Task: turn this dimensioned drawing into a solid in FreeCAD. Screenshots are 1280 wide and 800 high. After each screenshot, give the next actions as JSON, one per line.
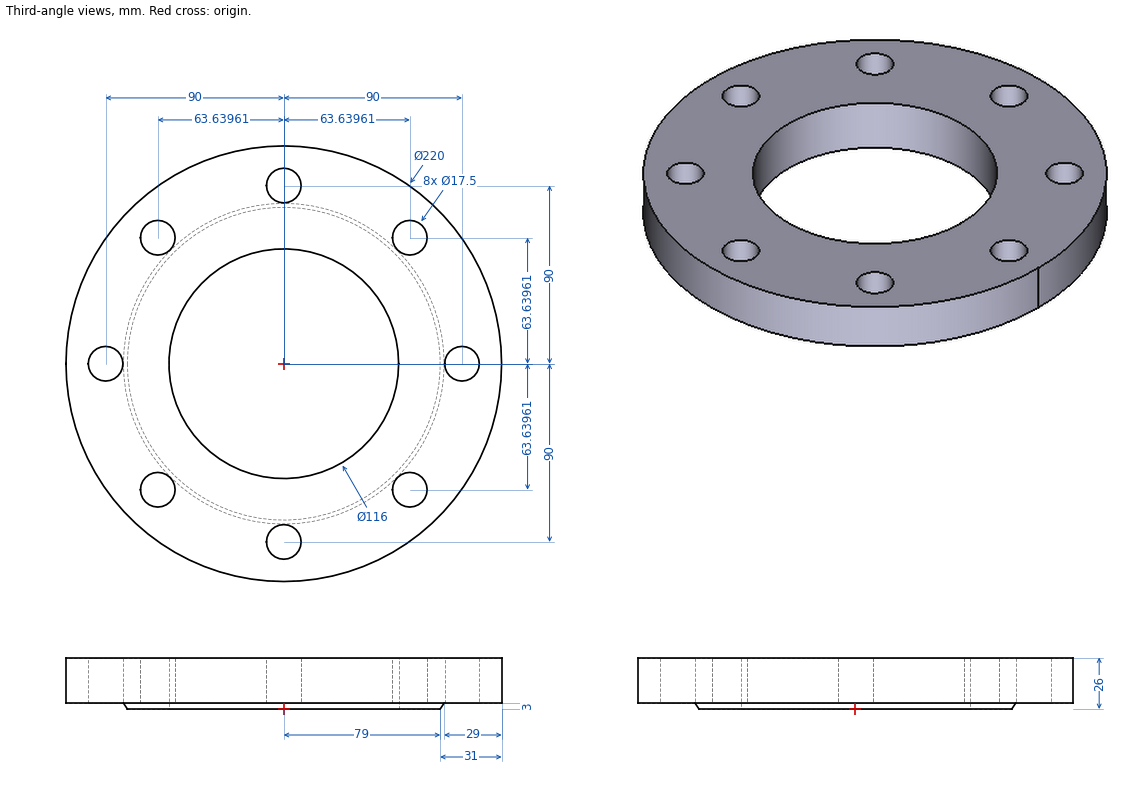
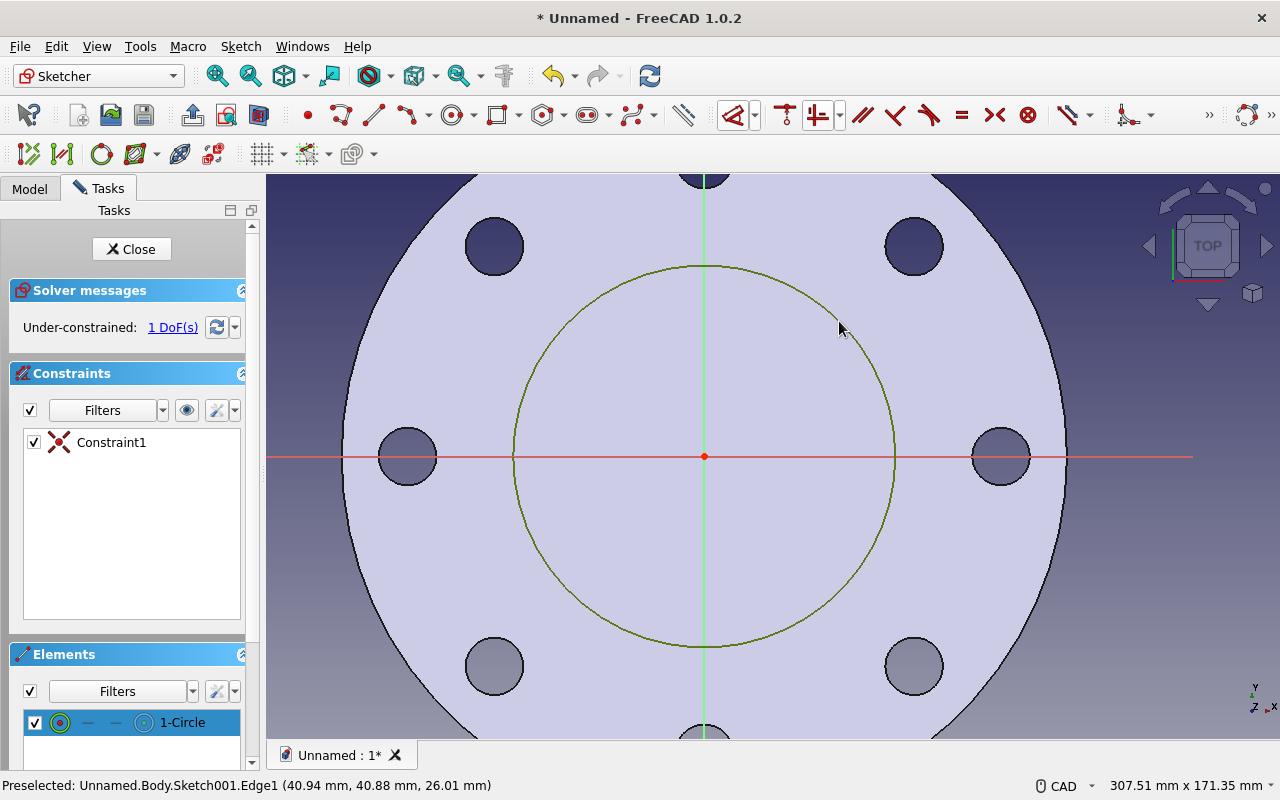
{"action": "left_click", "coordinate": [754, 116]}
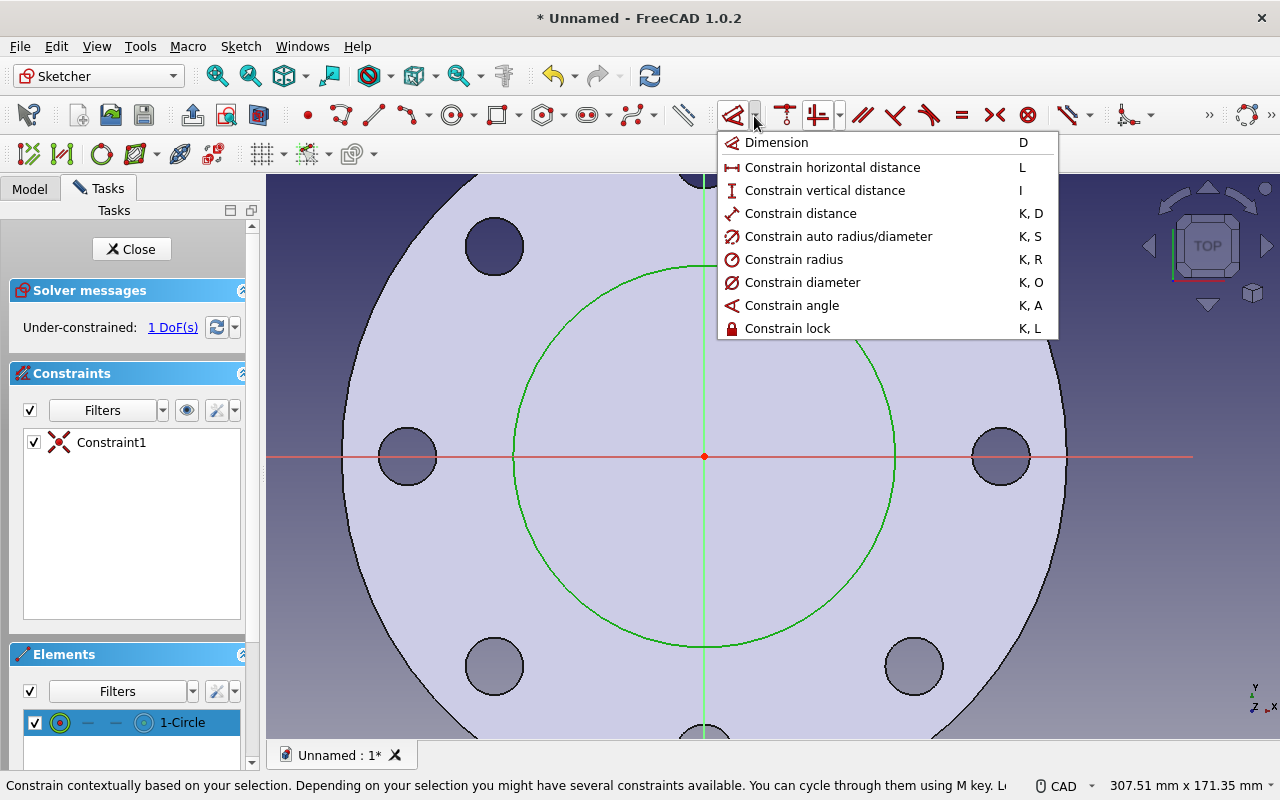
{"action": "left_click", "coordinate": [888, 282]}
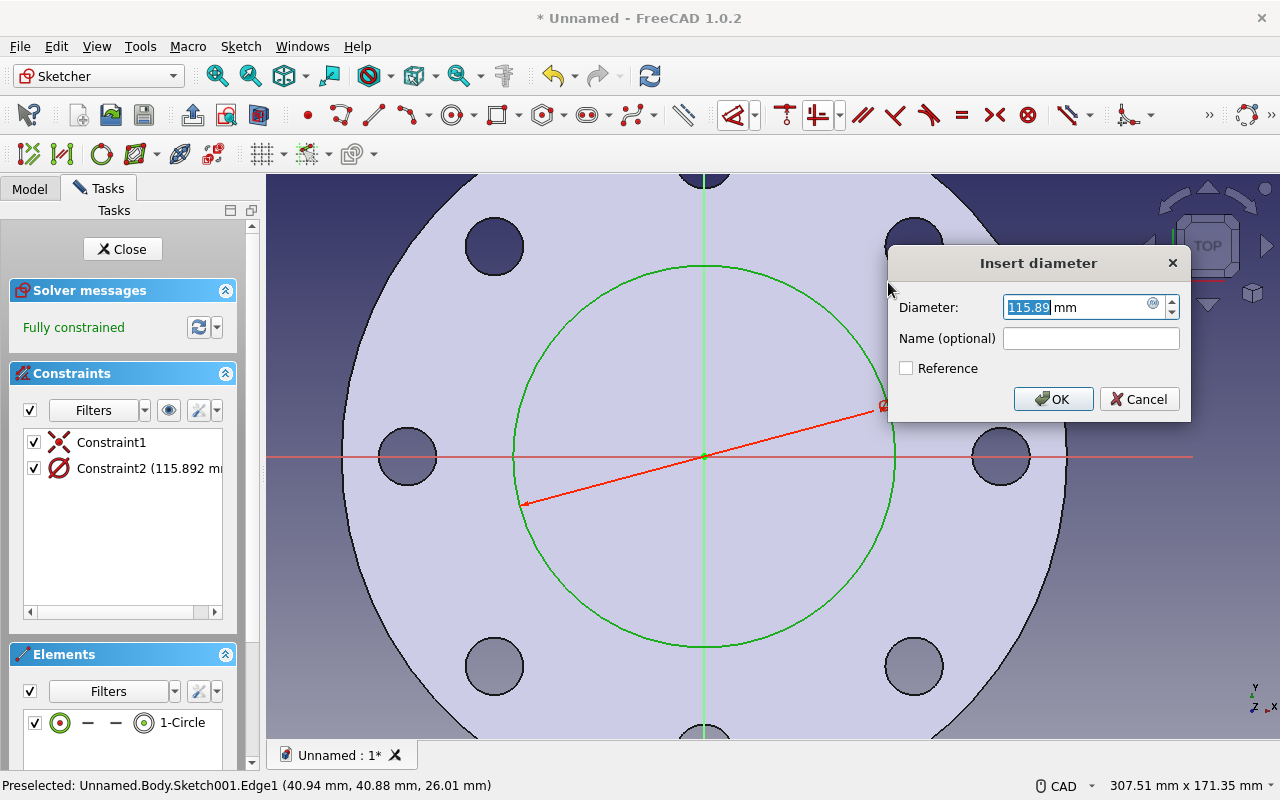
{"action": "type", "text": "116"}
{"action": "key", "text": "Return"}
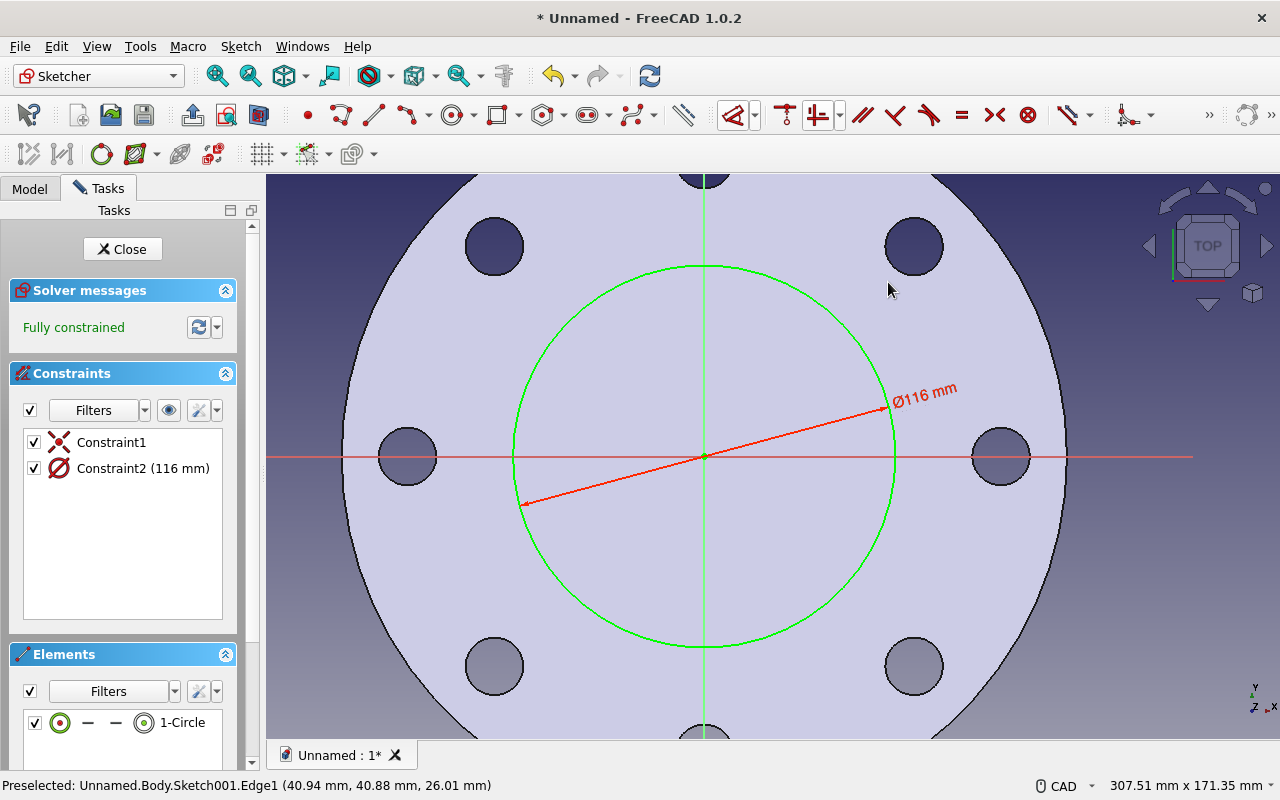
{"action": "left_click", "coordinate": [123, 249]}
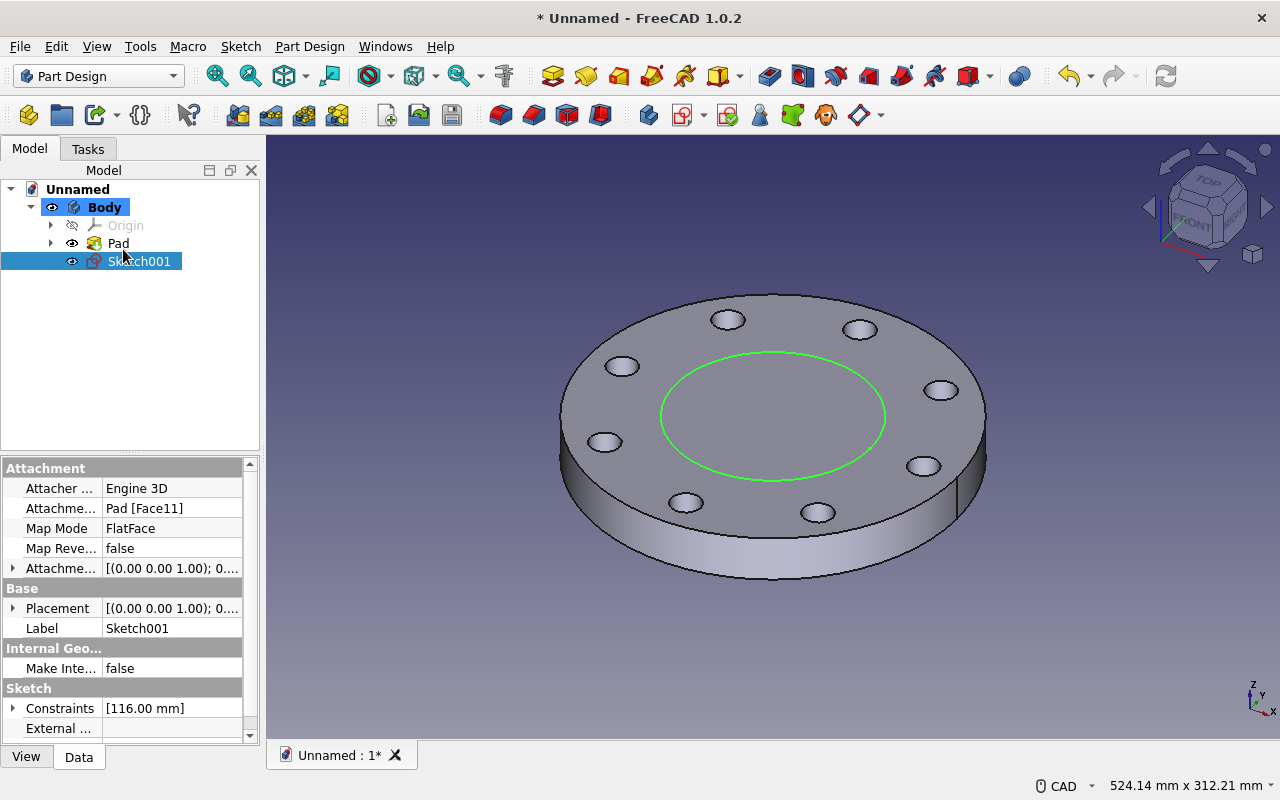
{"action": "left_click", "coordinate": [770, 76]}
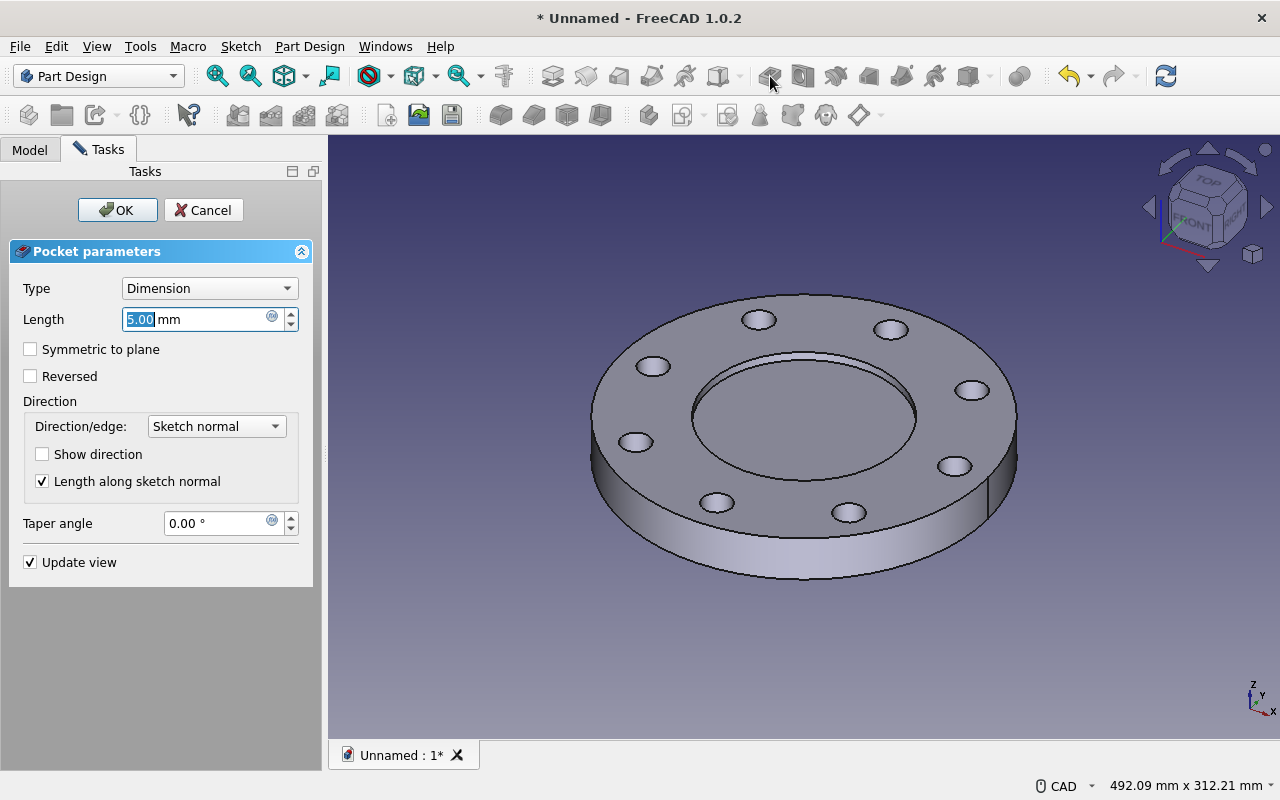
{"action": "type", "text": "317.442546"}
{"action": "key", "text": "Tab"}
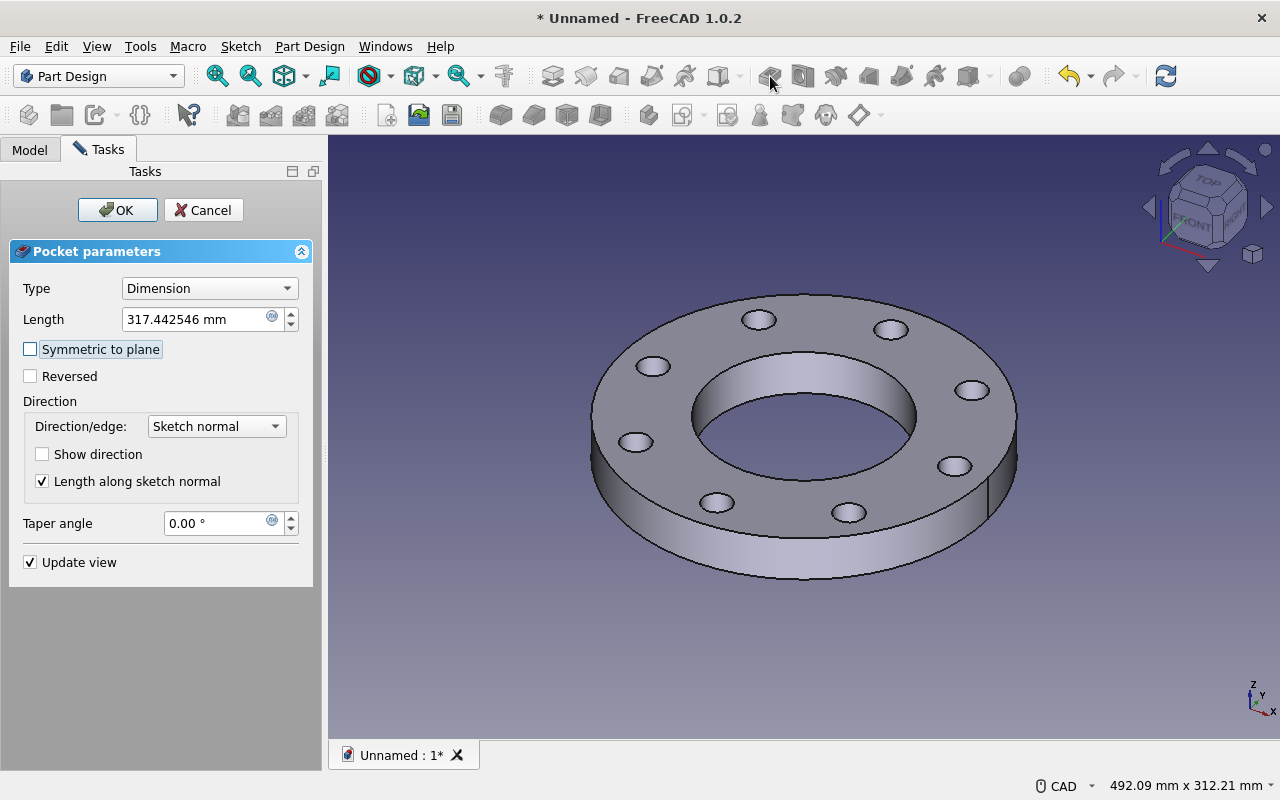
{"action": "left_click", "coordinate": [31, 349]}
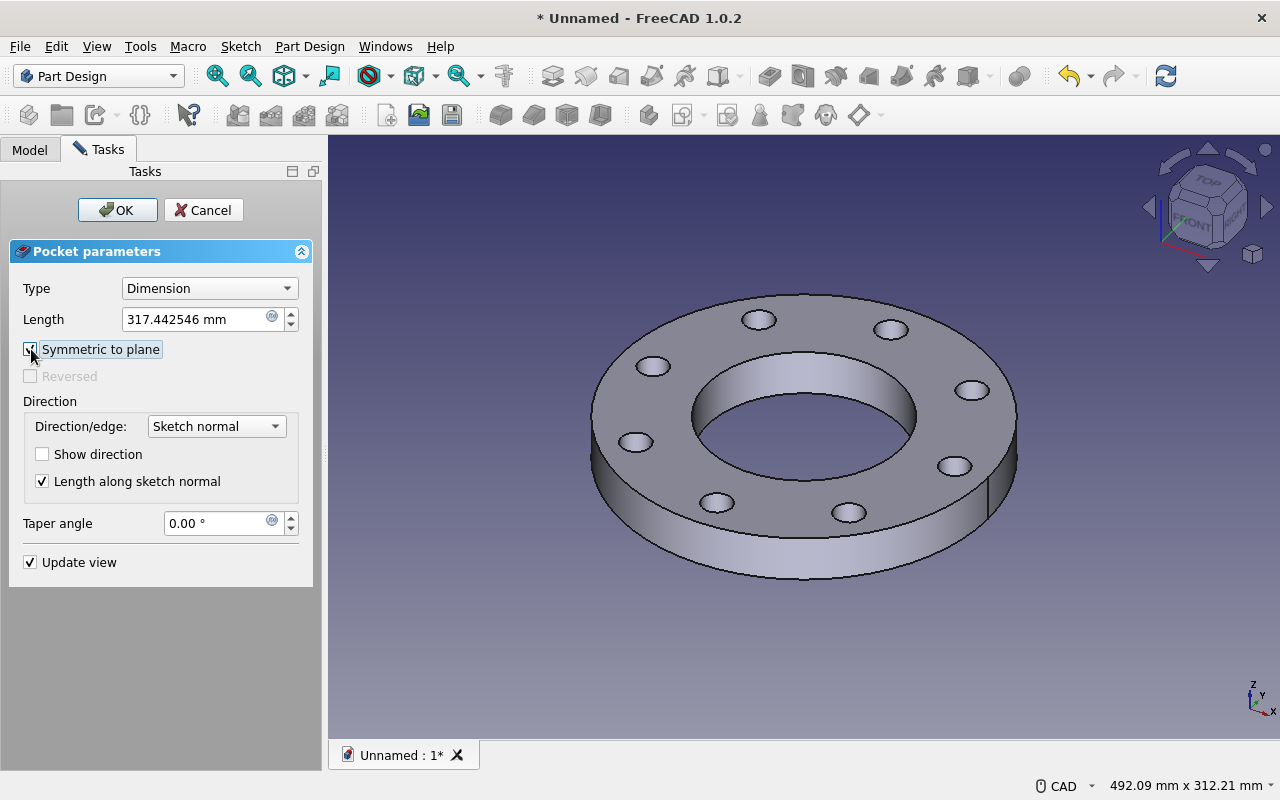
{"action": "left_click", "coordinate": [118, 210]}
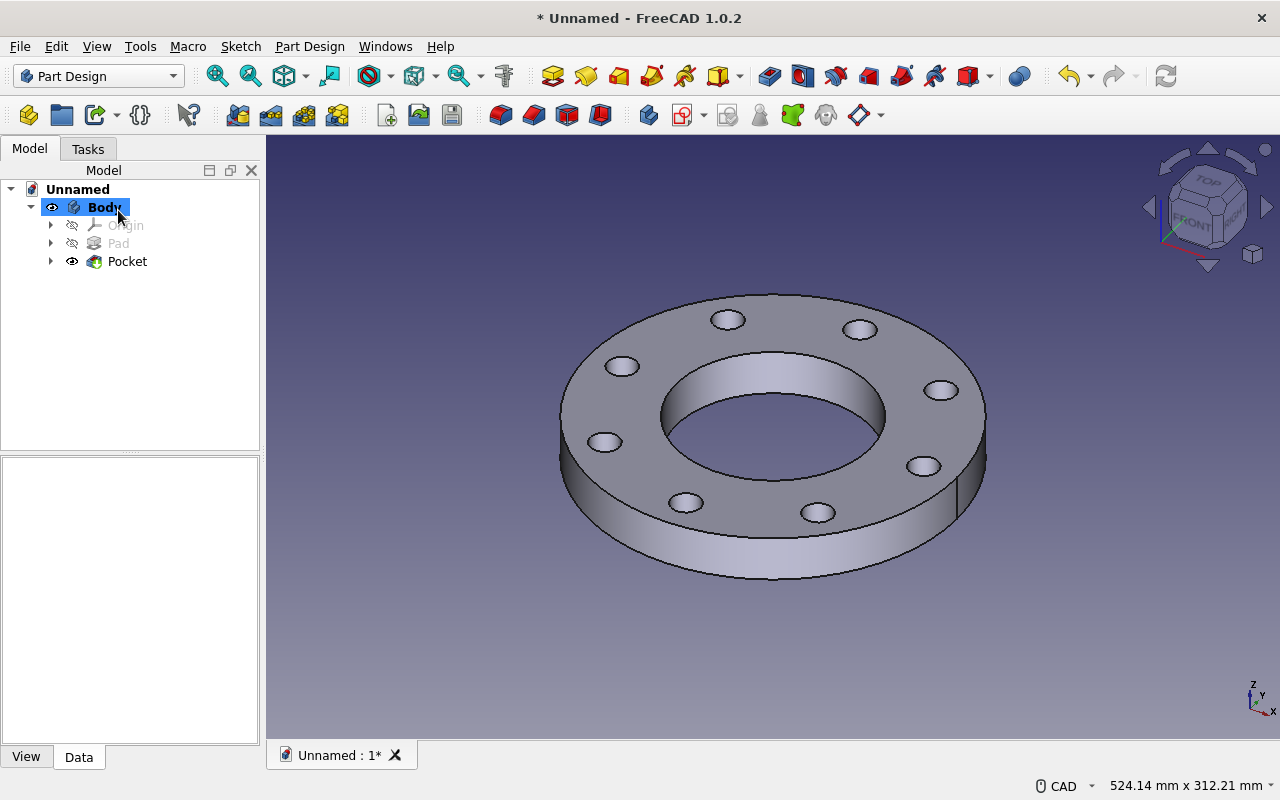
{"action": "left_click", "coordinate": [682, 116]}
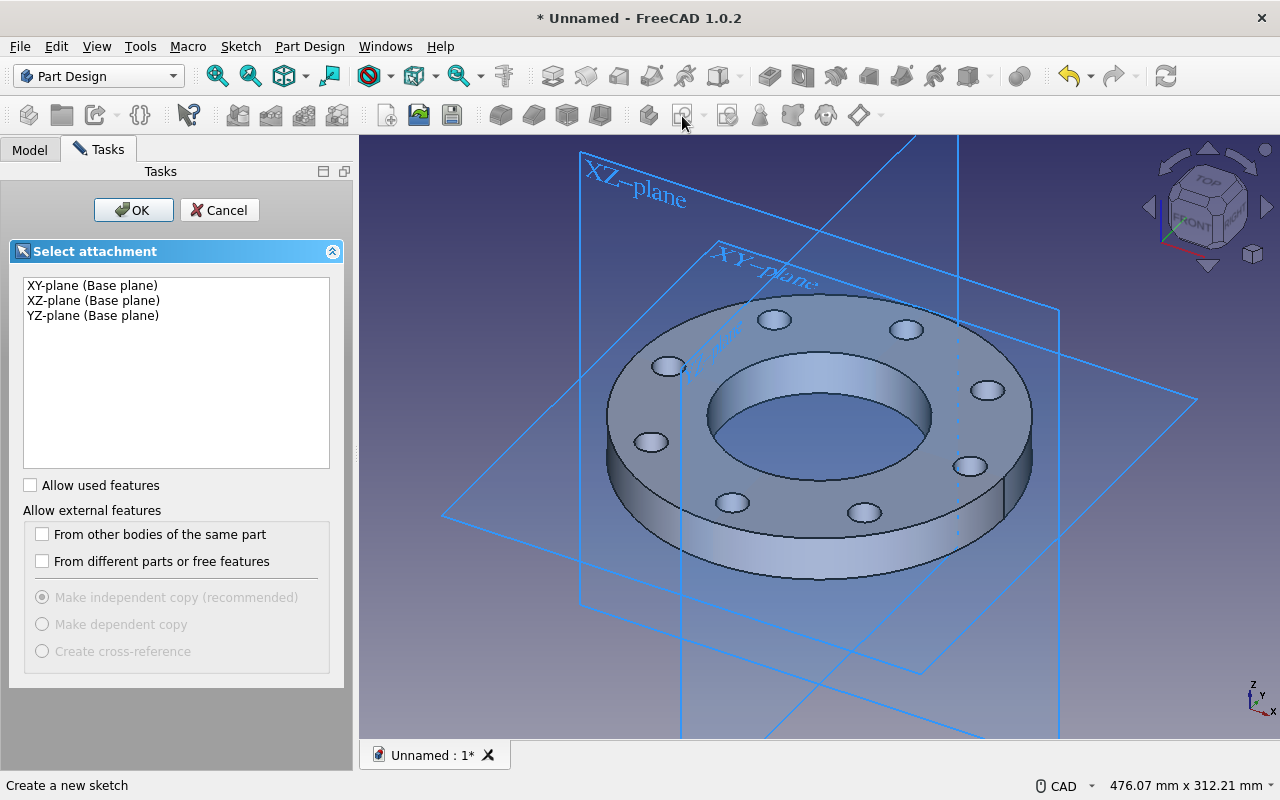
{"action": "left_click", "coordinate": [84, 300]}